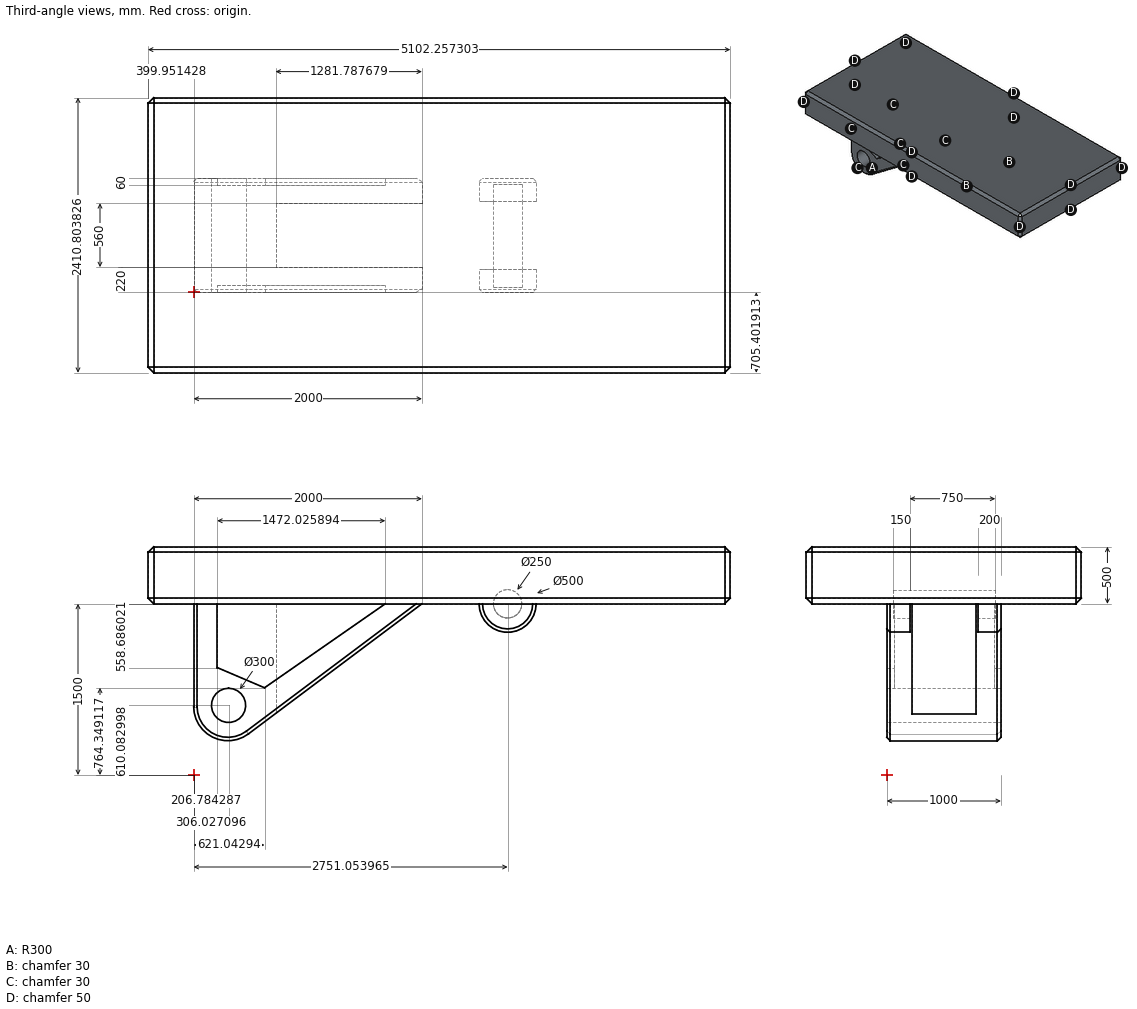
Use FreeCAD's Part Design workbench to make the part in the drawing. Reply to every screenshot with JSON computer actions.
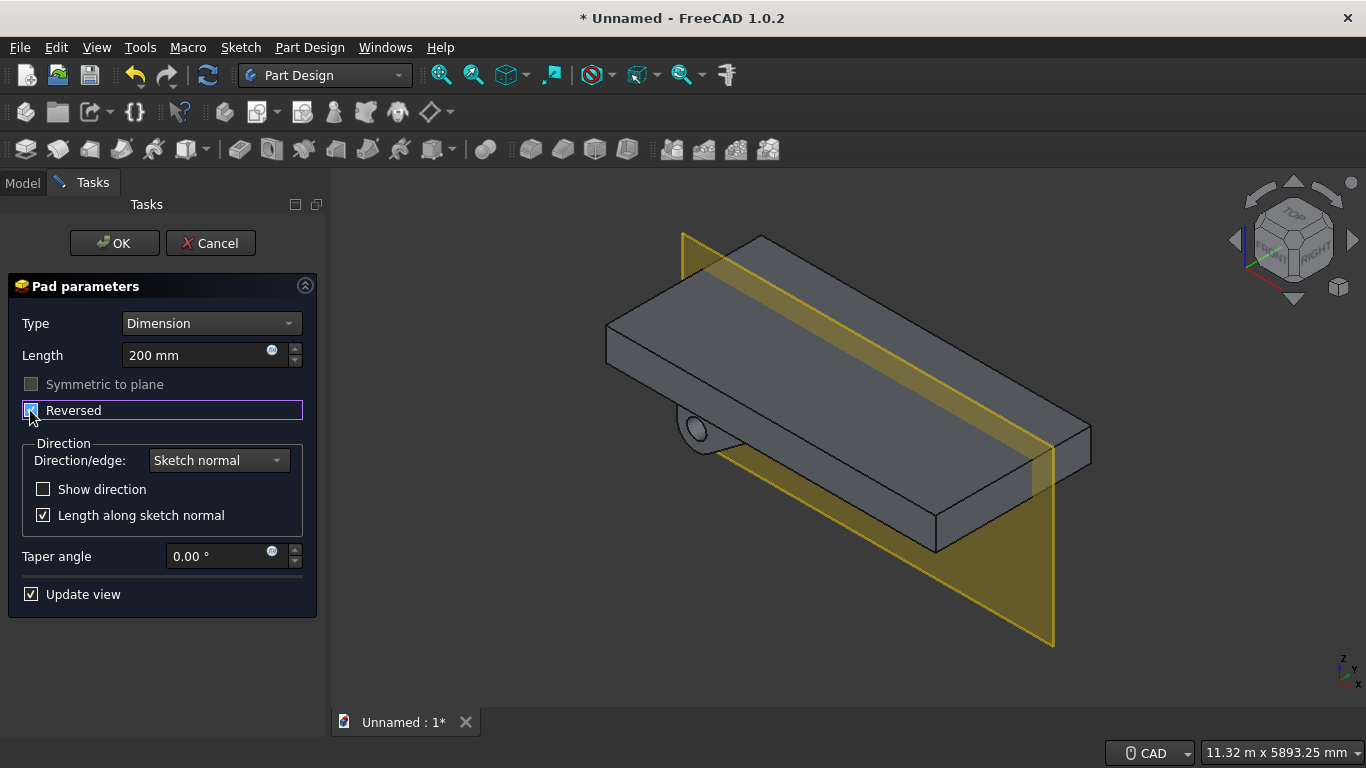
{"action": "left_click", "coordinate": [115, 243]}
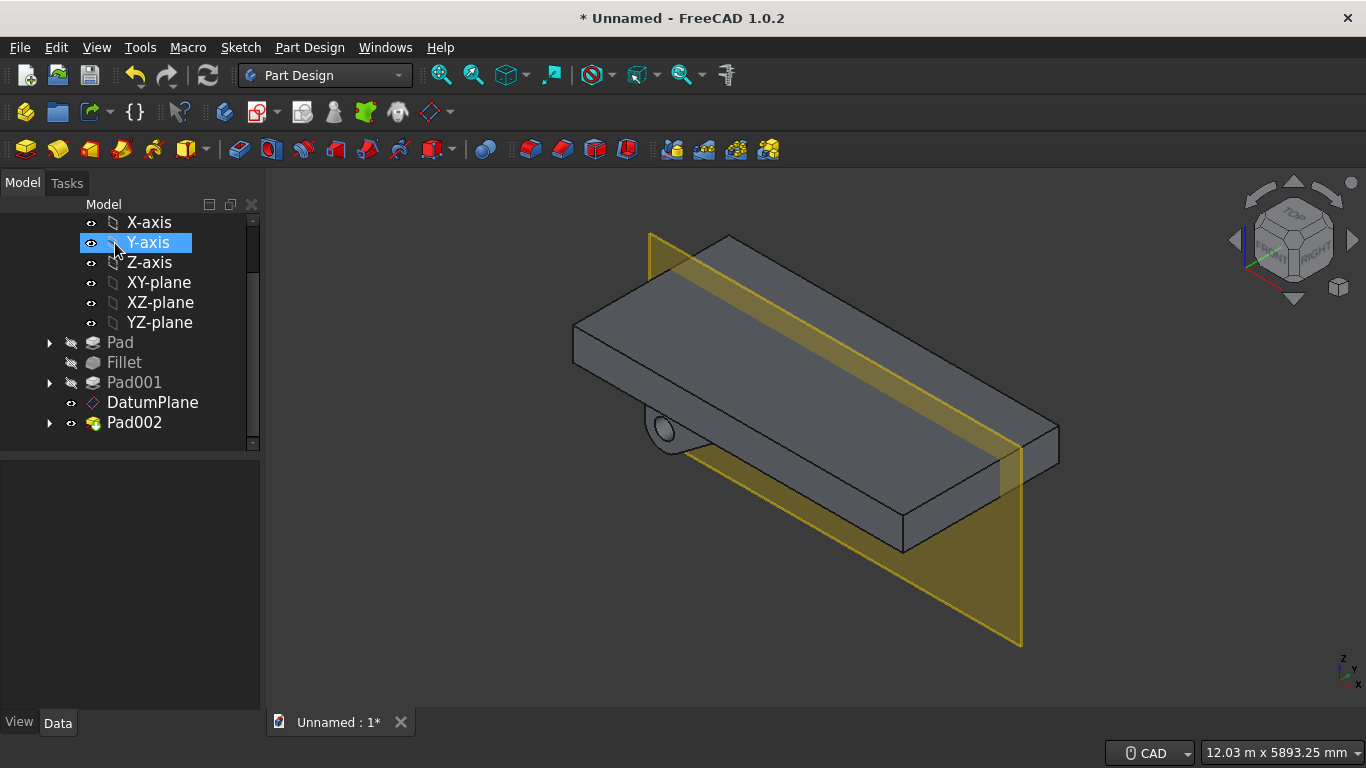
{"action": "left_click", "coordinate": [116, 403]}
{"action": "key", "text": "space"}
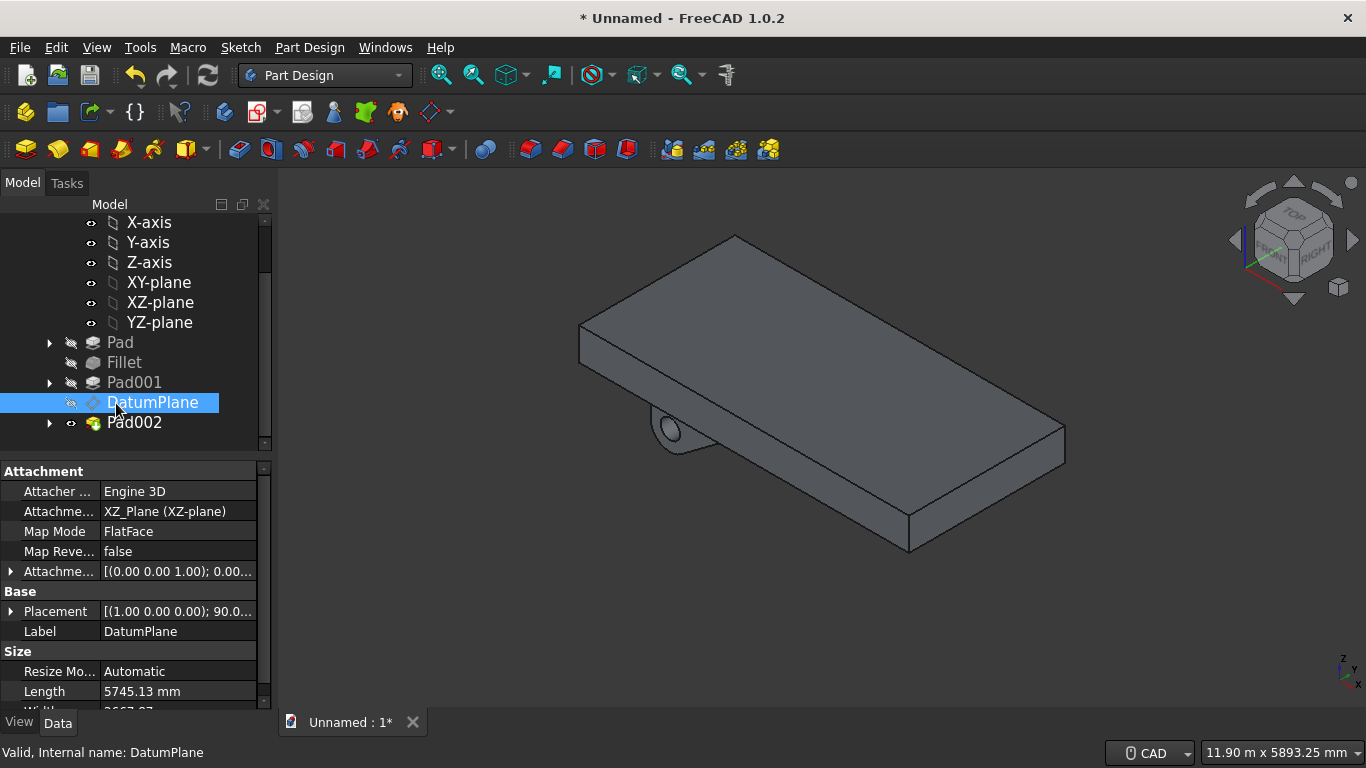
{"action": "scroll", "coordinate": [160, 318], "scroll_direction": "down", "scroll_amount": 3}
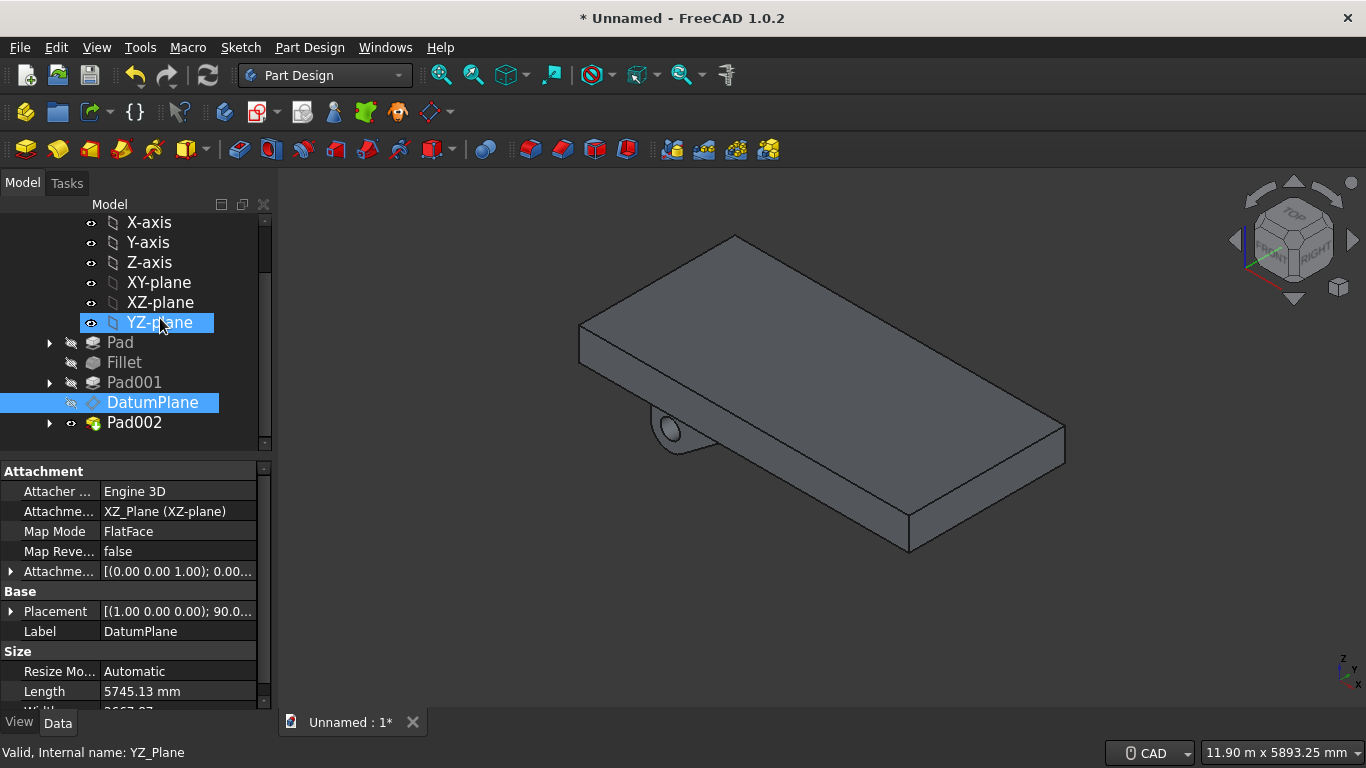
{"action": "scroll", "coordinate": [160, 318], "scroll_direction": "up", "scroll_amount": 15}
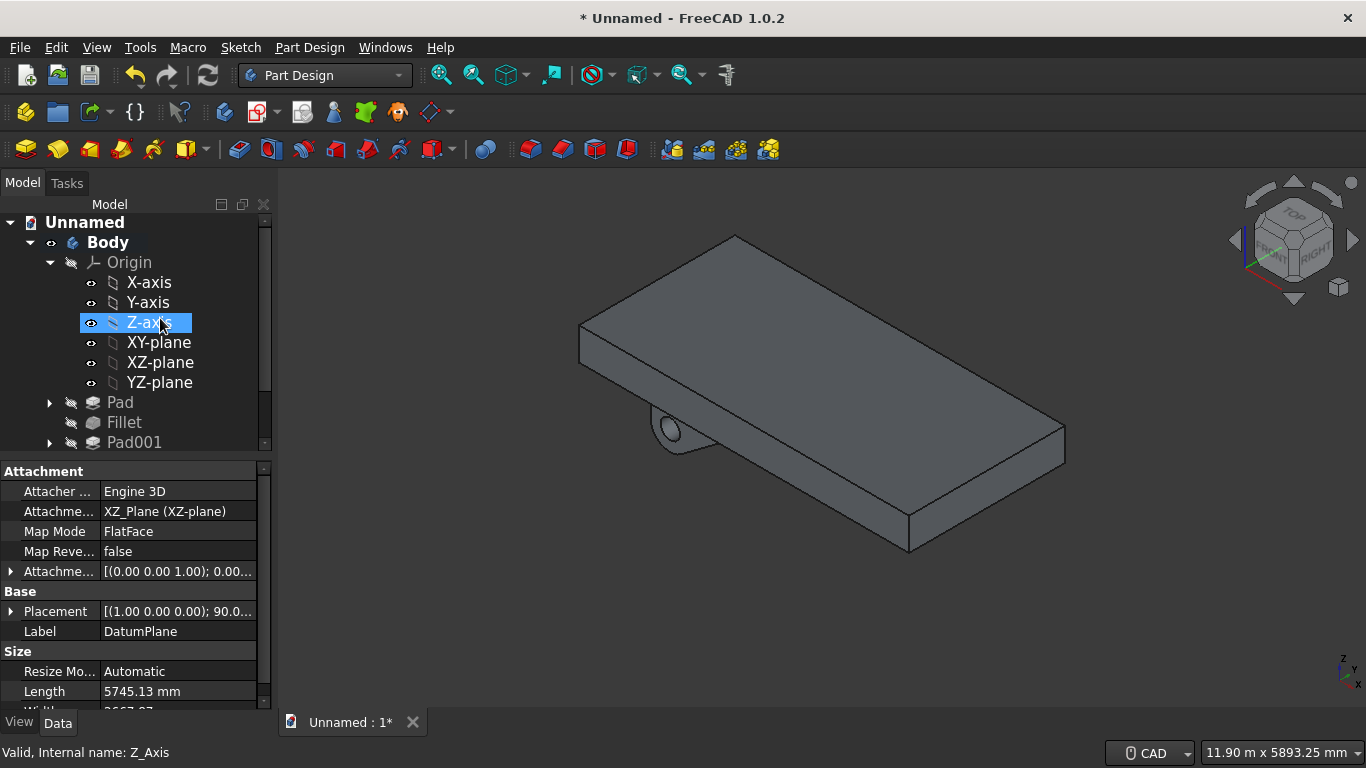
{"action": "left_click", "coordinate": [136, 363]}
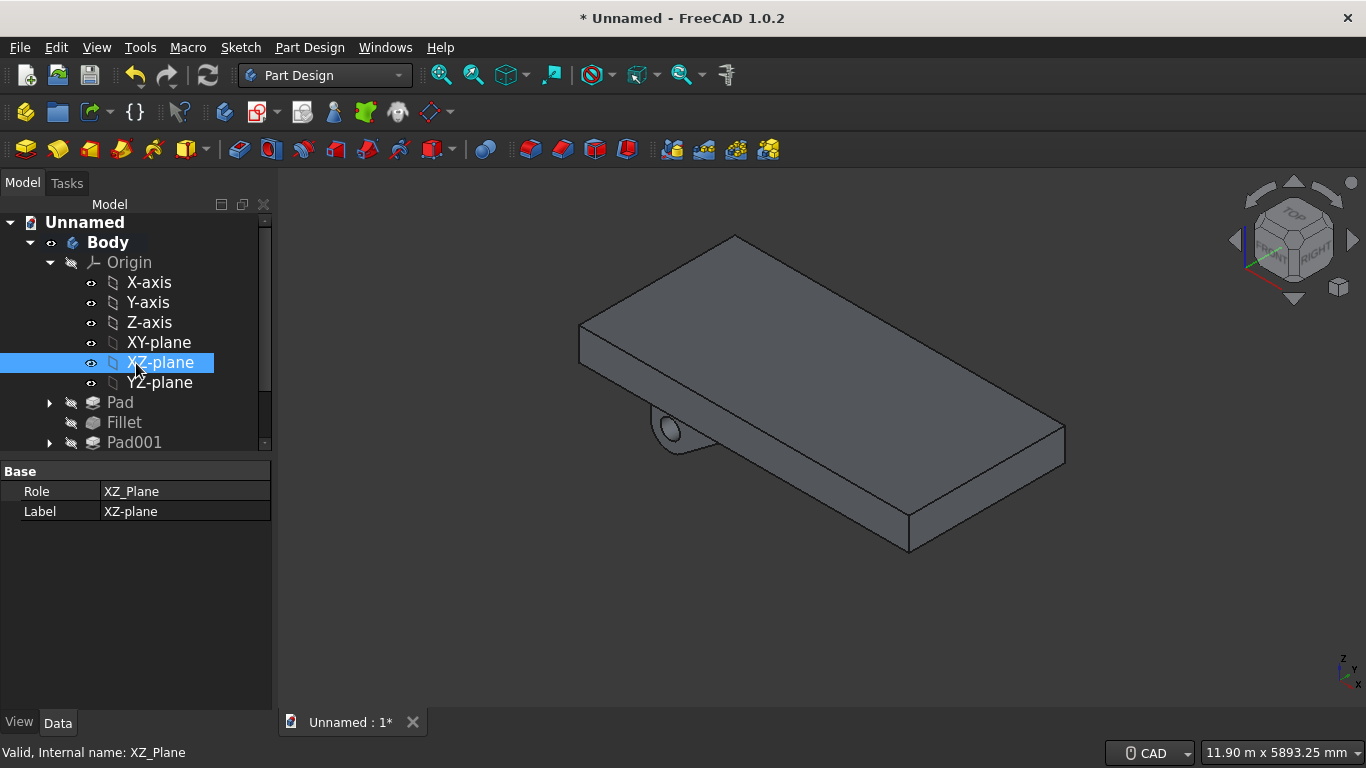
{"action": "left_click", "coordinate": [430, 112]}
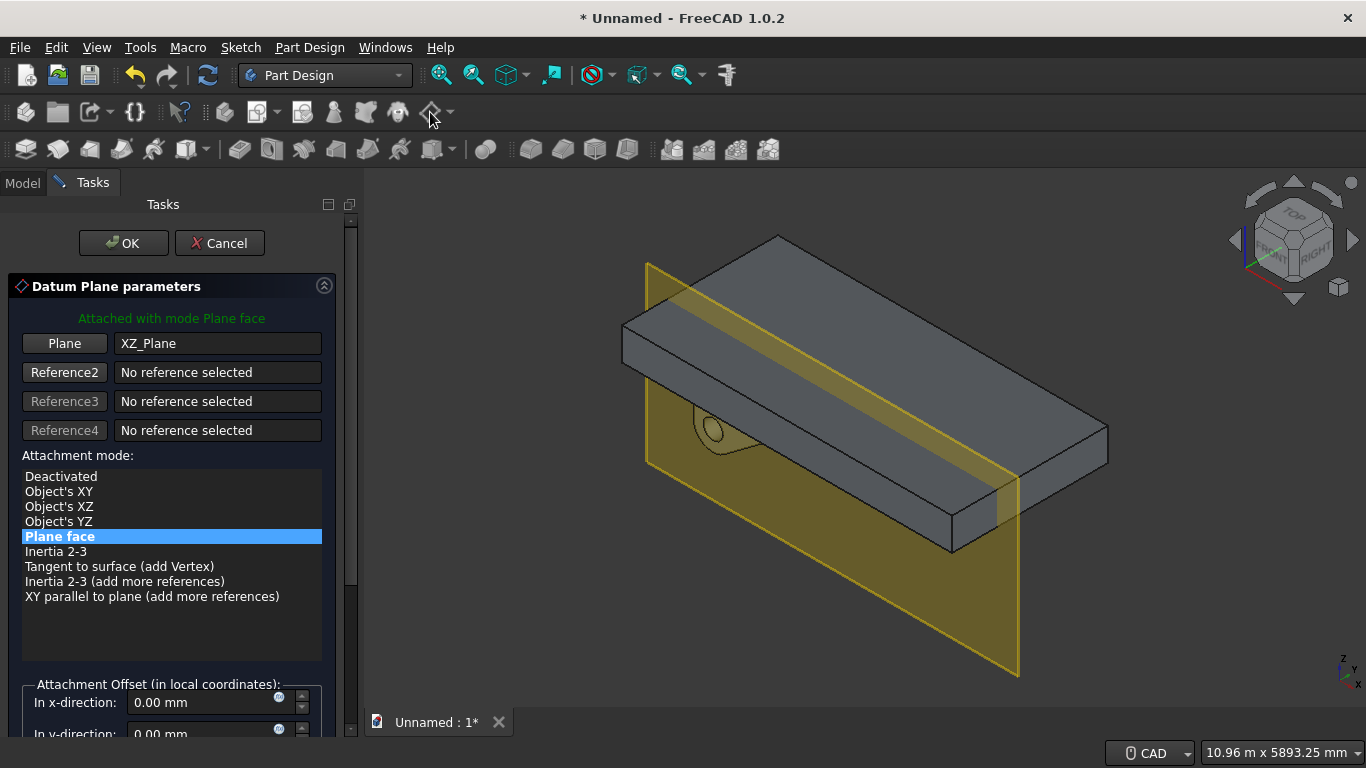
{"action": "scroll", "coordinate": [351, 475], "scroll_direction": "down", "scroll_amount": 2}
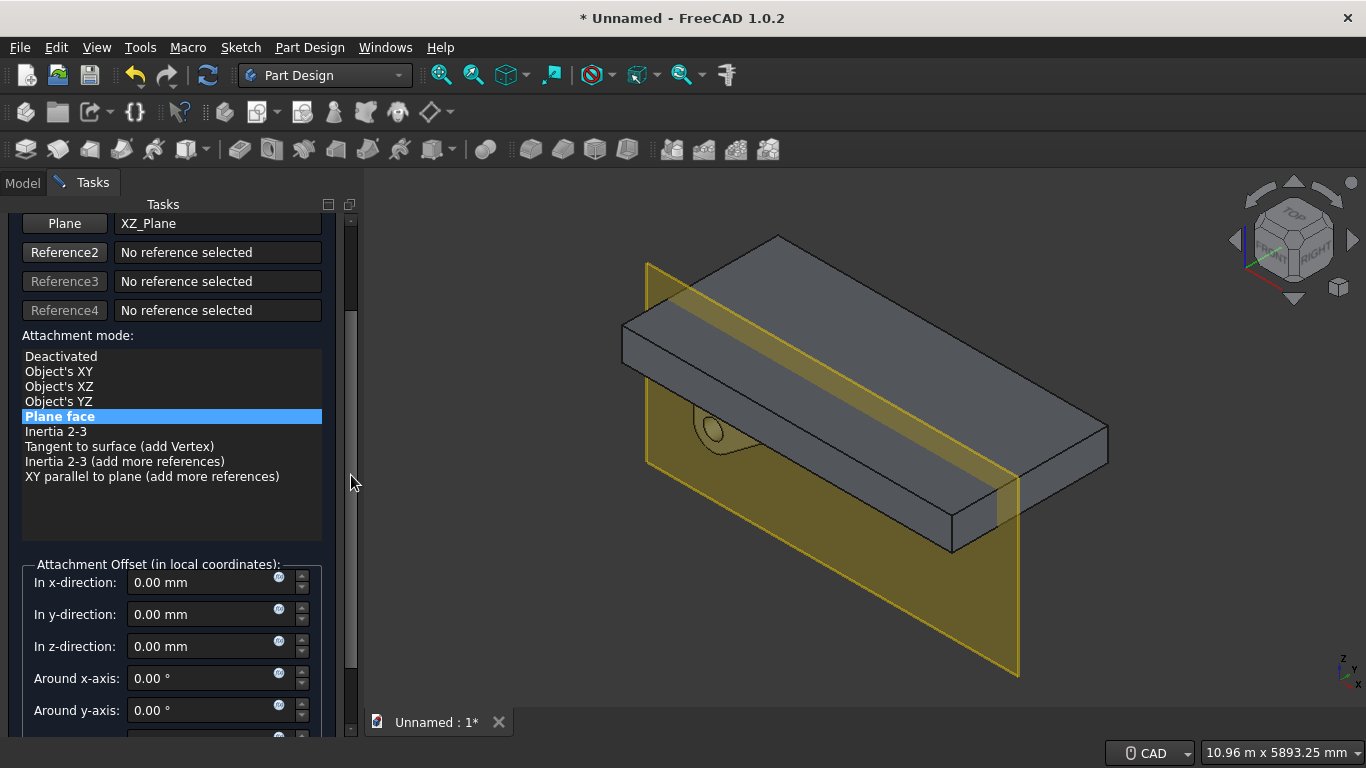
{"action": "triple_click", "coordinate": [210, 646]}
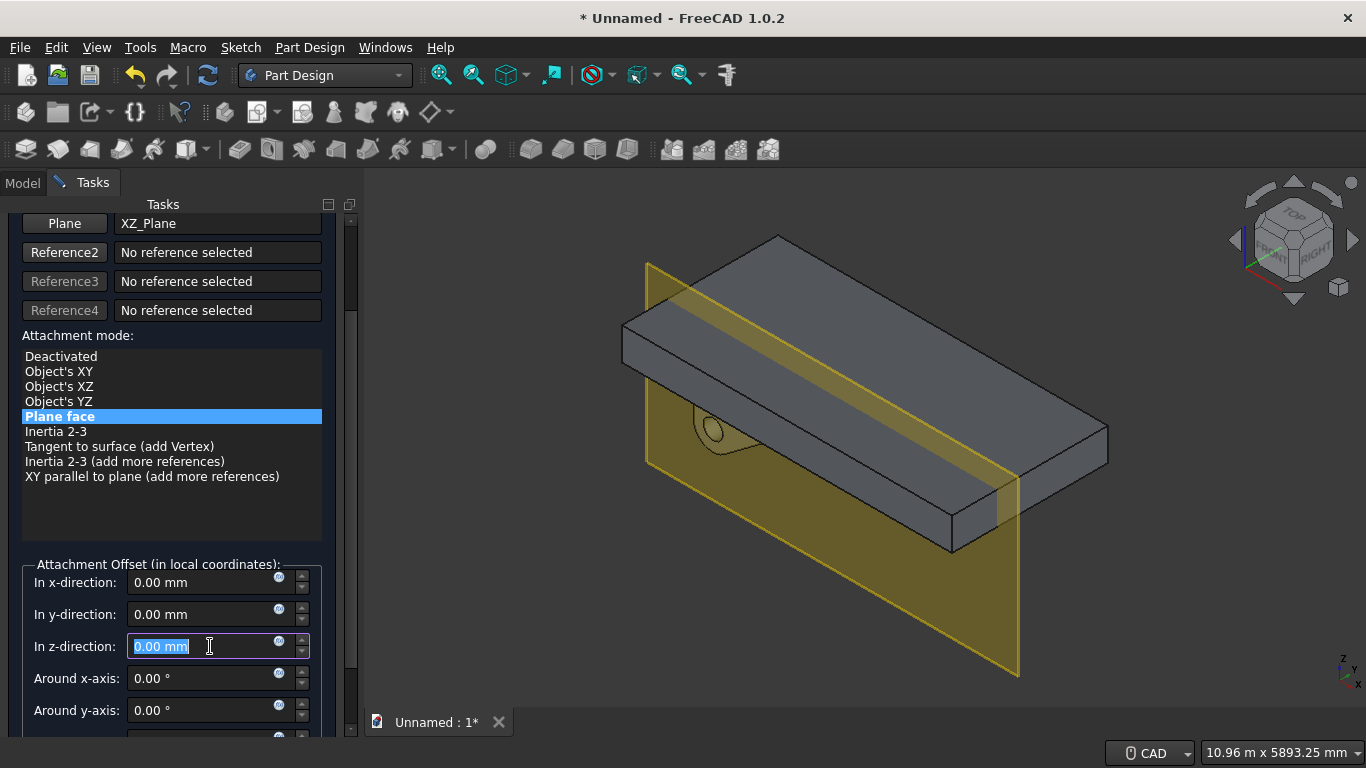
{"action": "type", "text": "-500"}
{"action": "key", "text": "Tab"}